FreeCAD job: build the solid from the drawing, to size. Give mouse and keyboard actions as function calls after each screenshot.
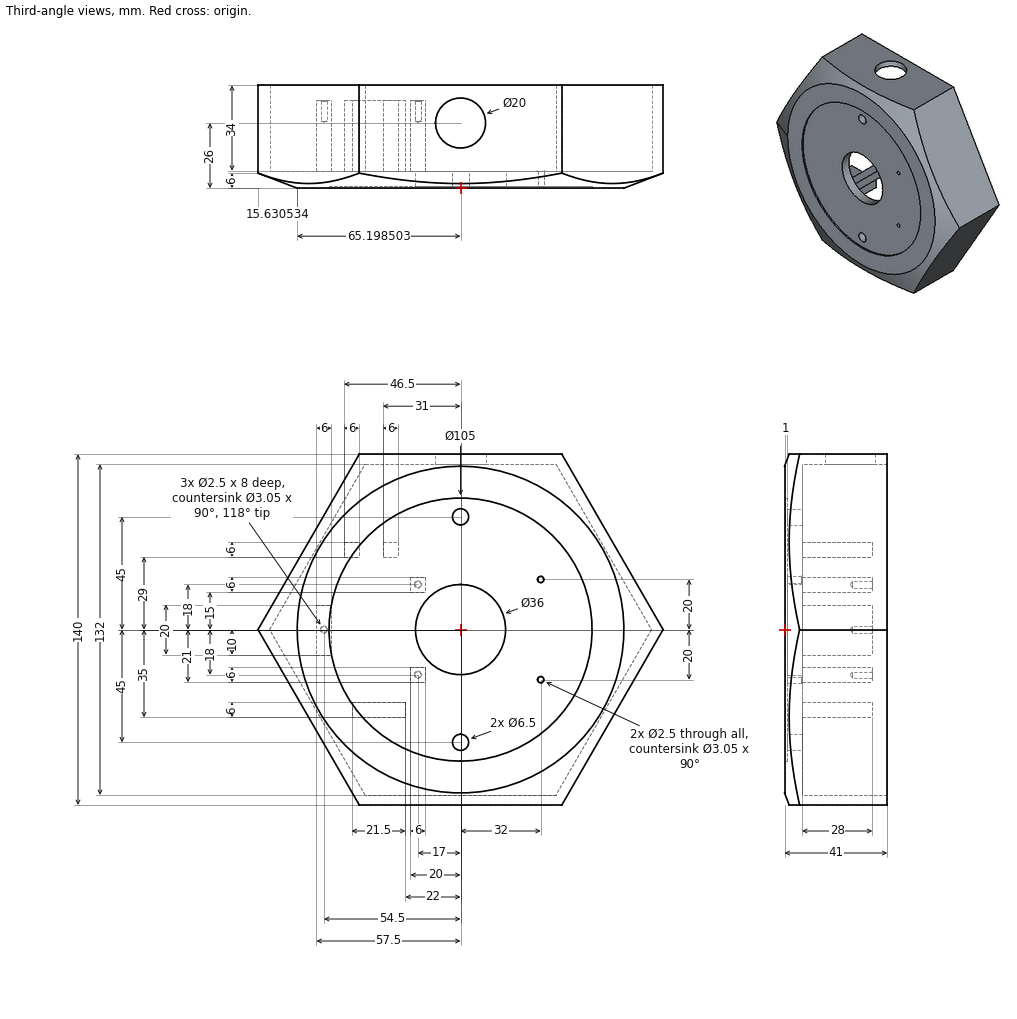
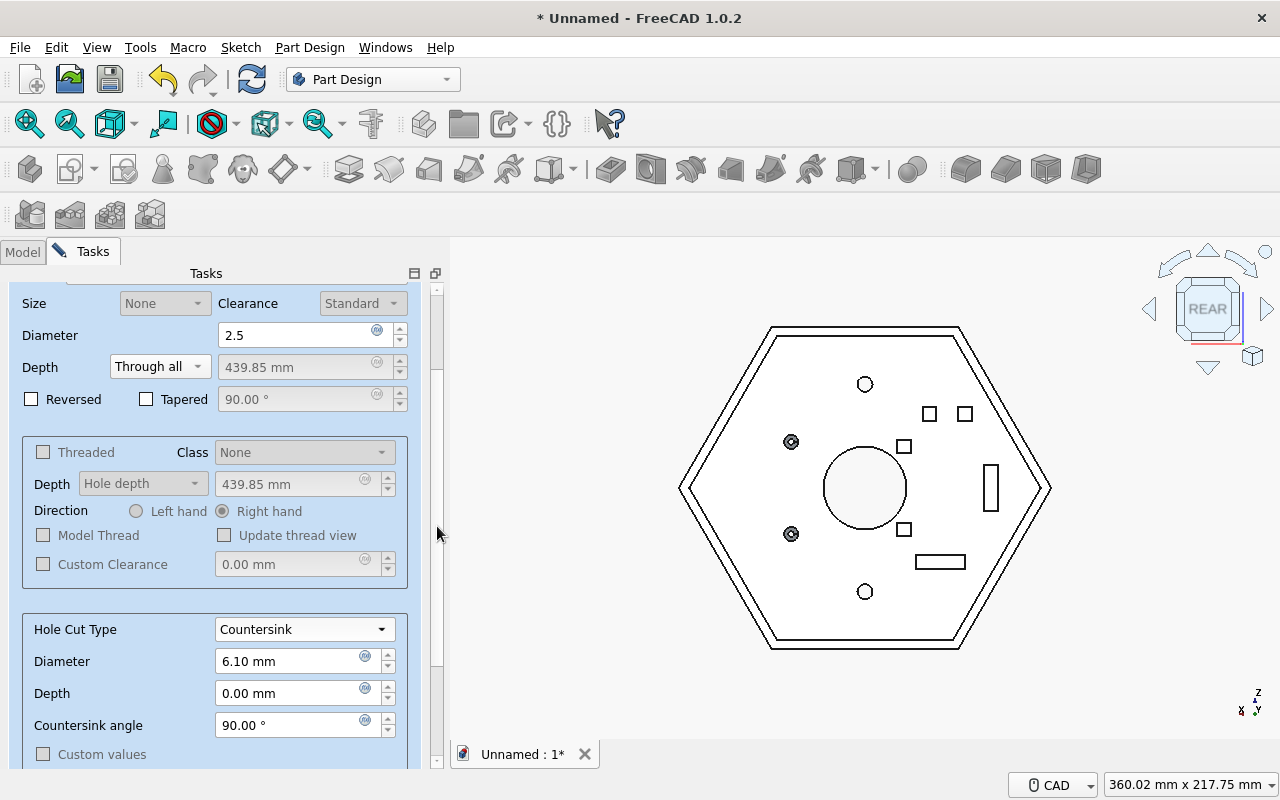
triple_click(298, 661)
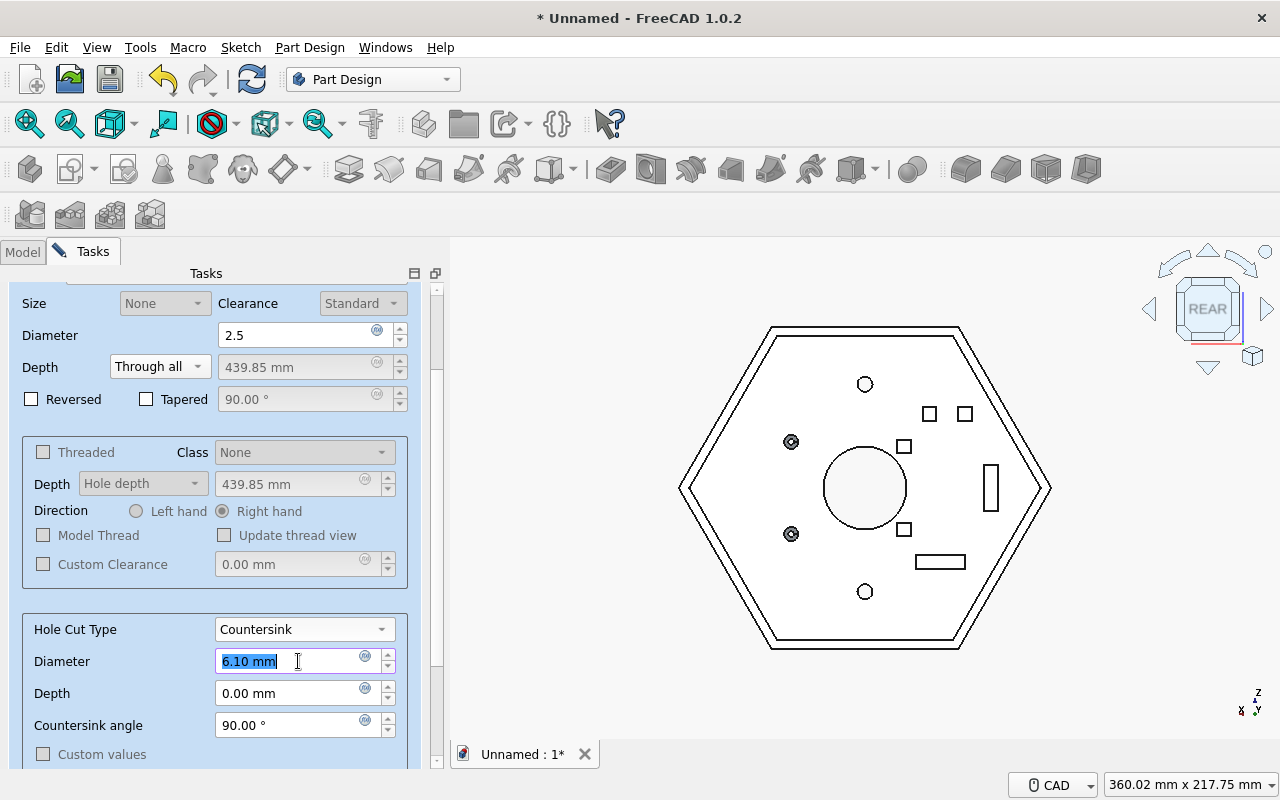
text(3.05)
key(Tab)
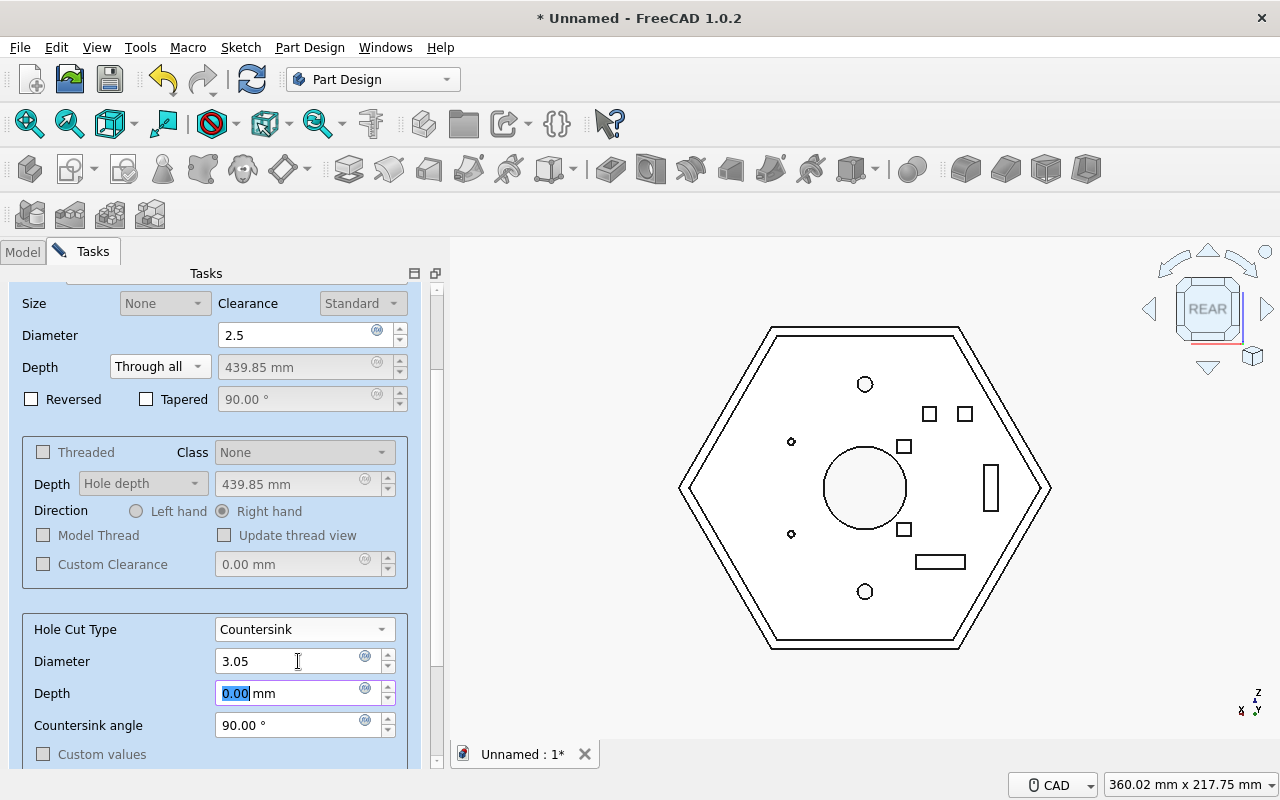
scroll(437, 526, up, 3)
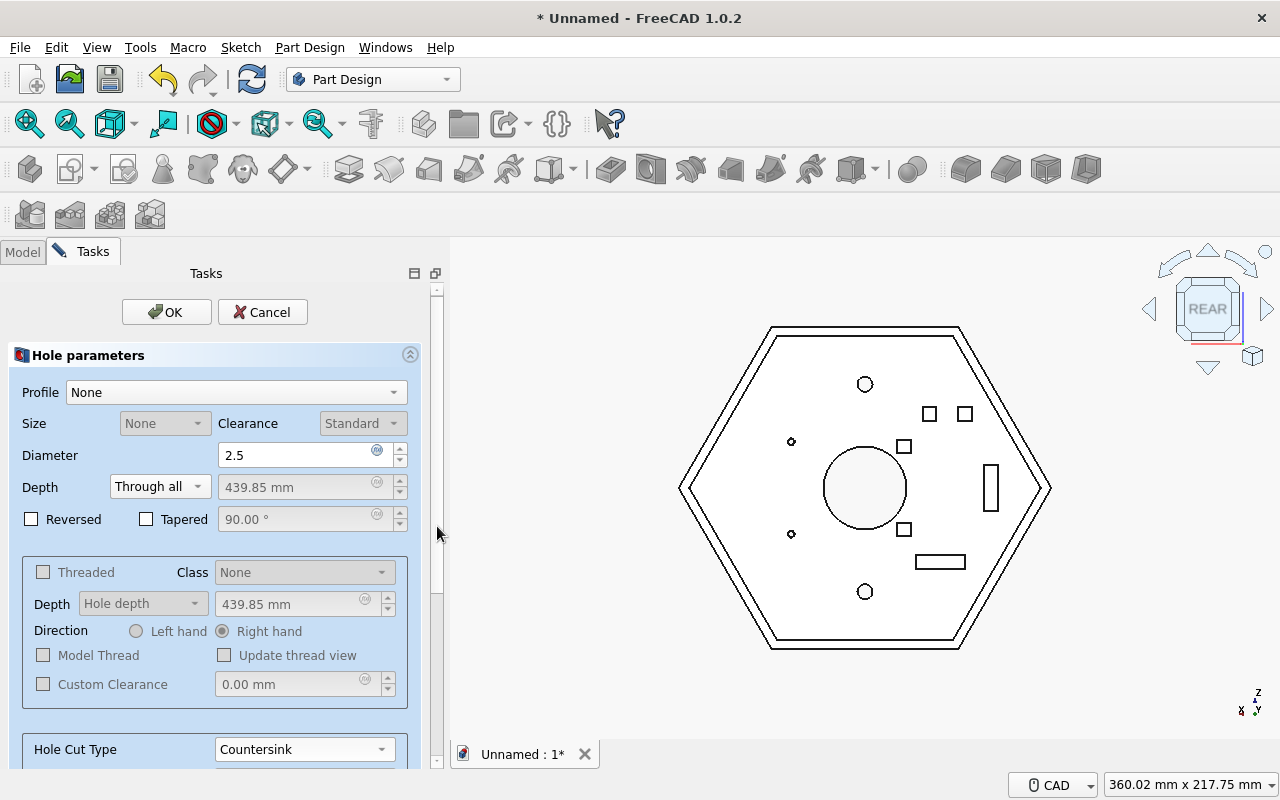
click(167, 312)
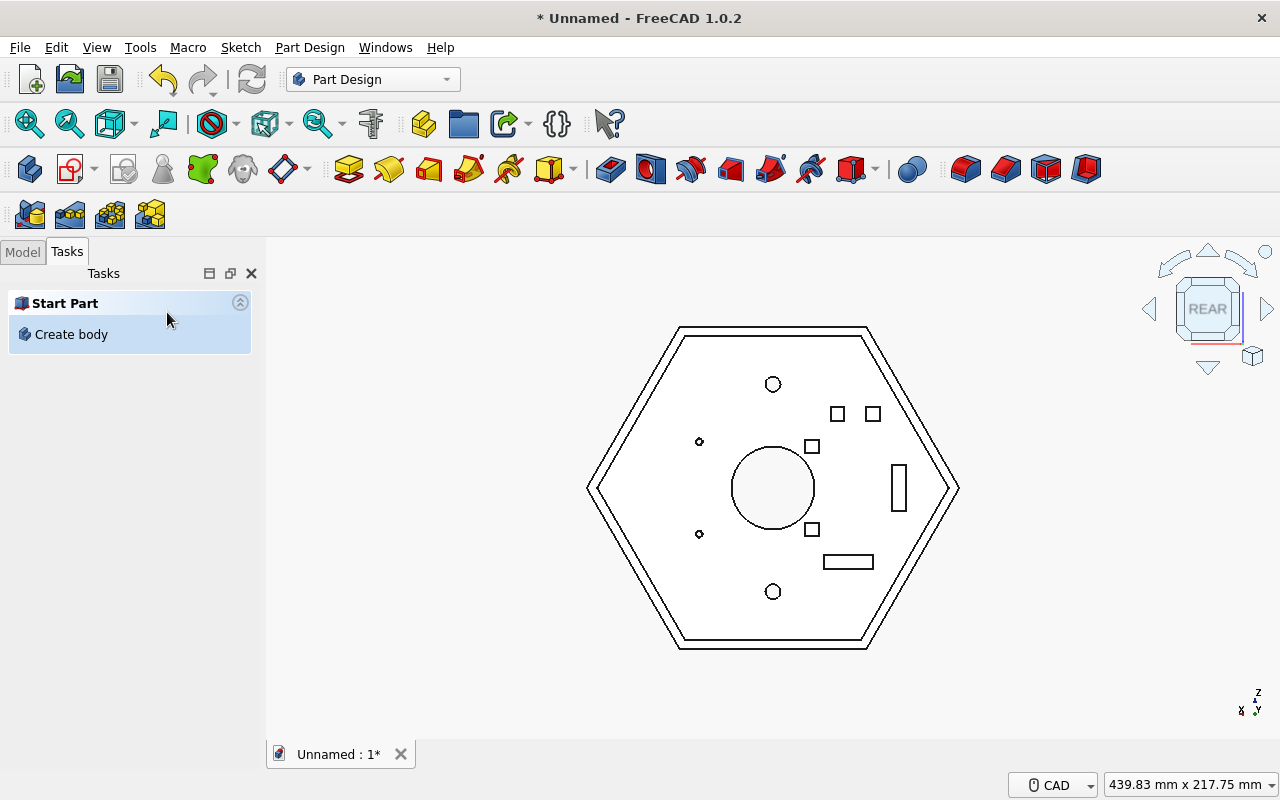
click(834, 559)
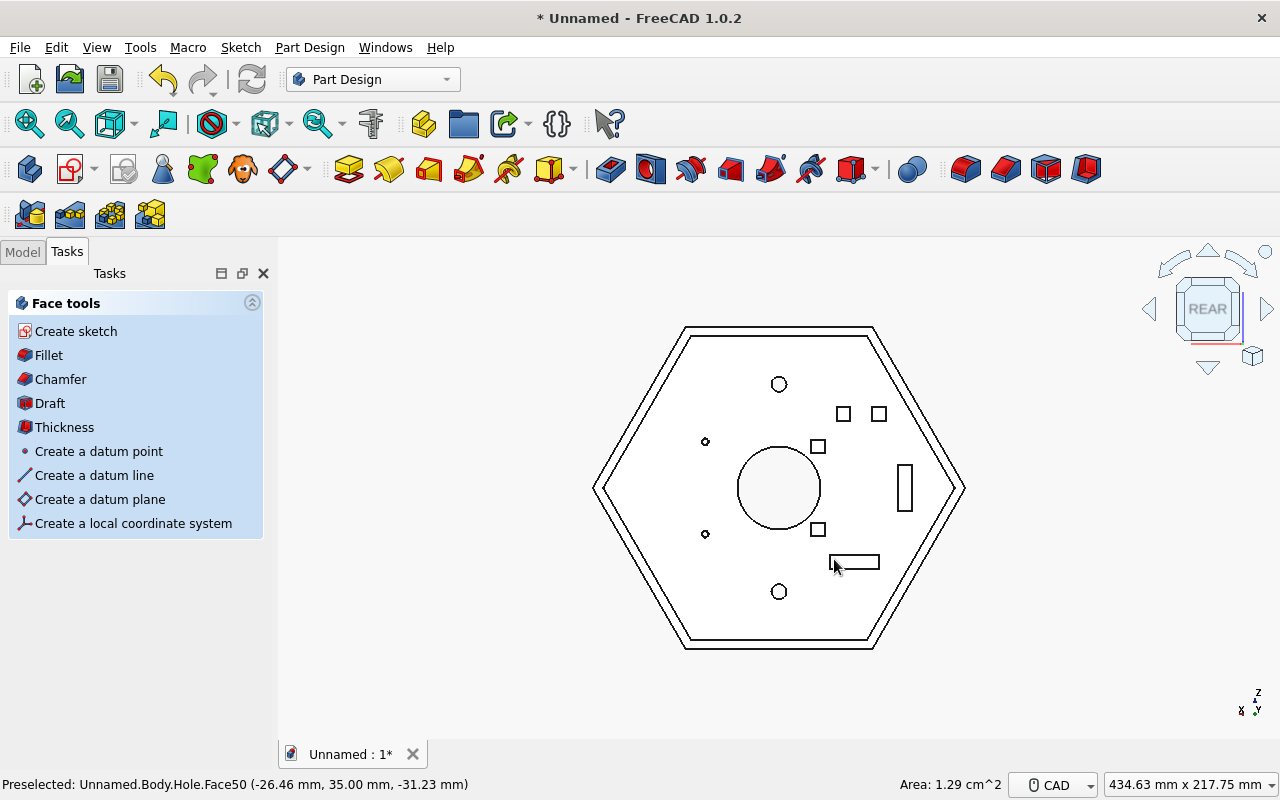
click(70, 170)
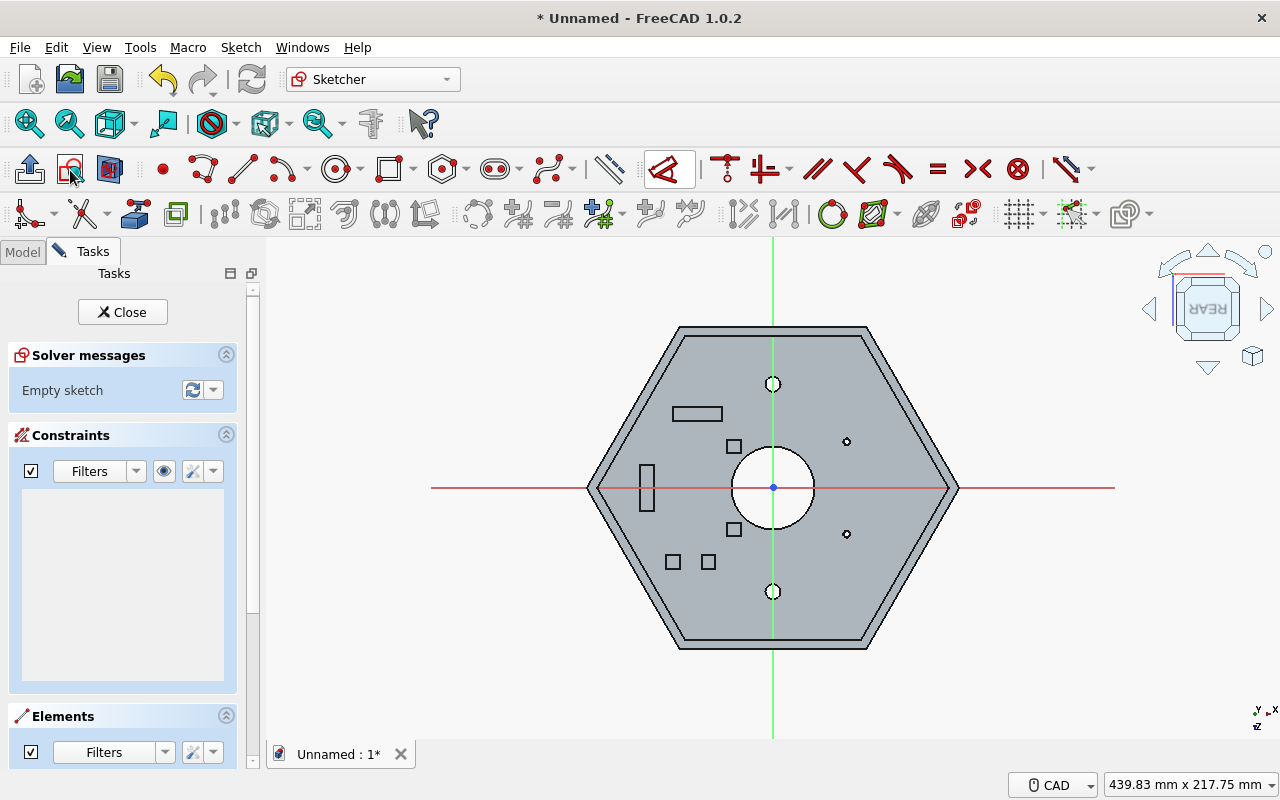
scroll(711, 488, up, 6)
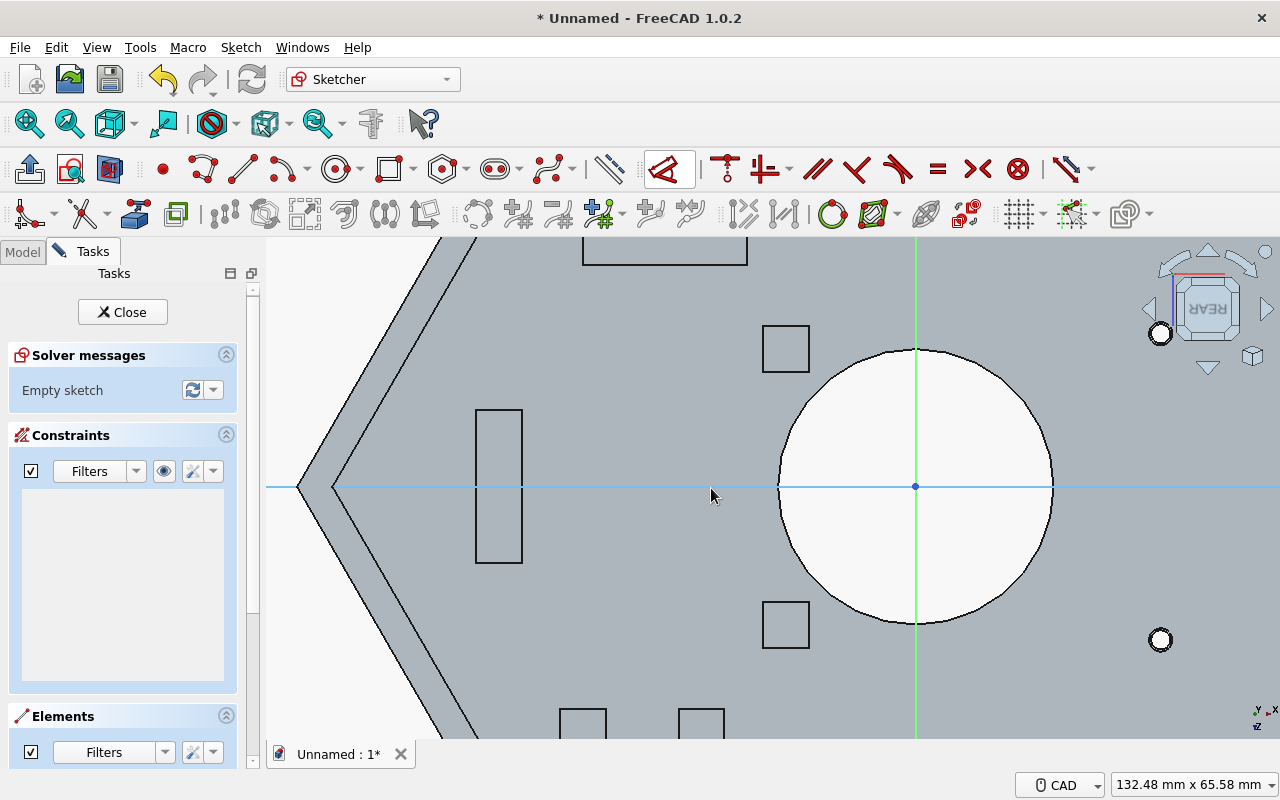
click(336, 170)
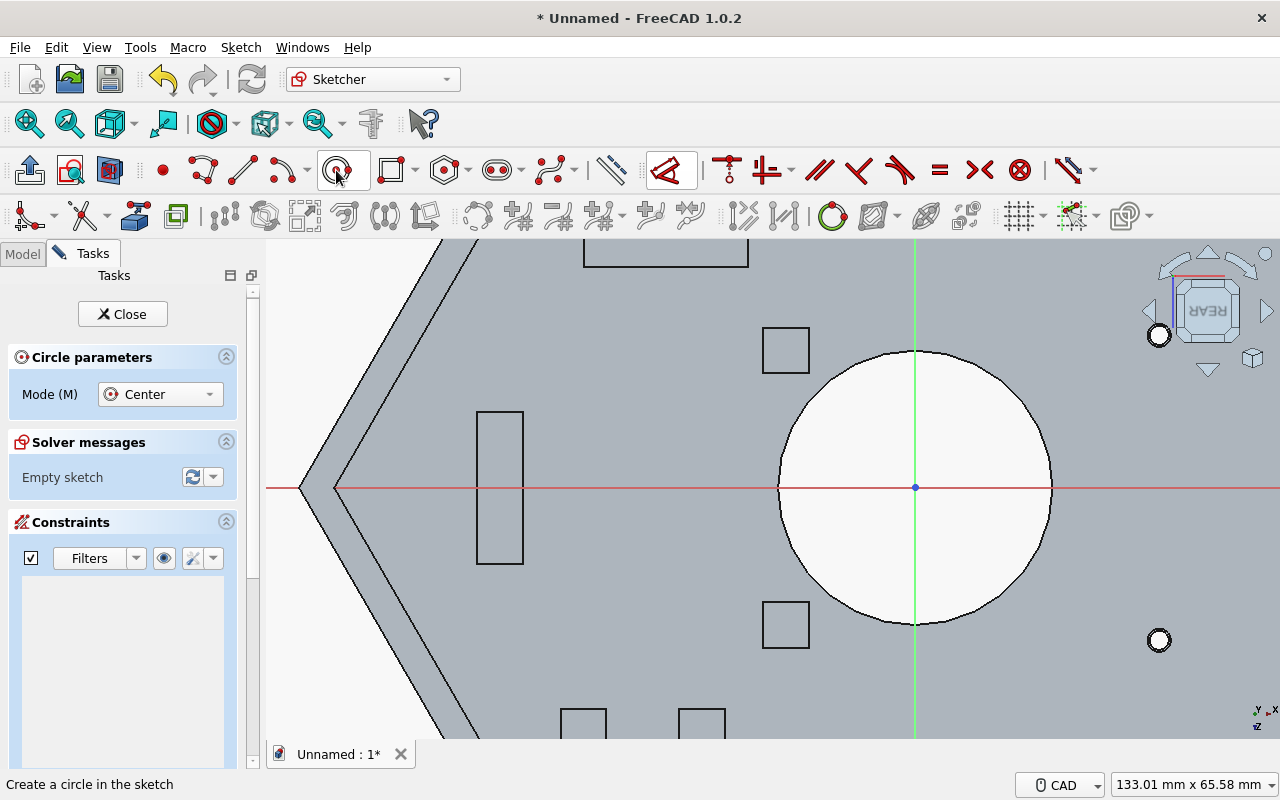
scroll(500, 488, up, 5)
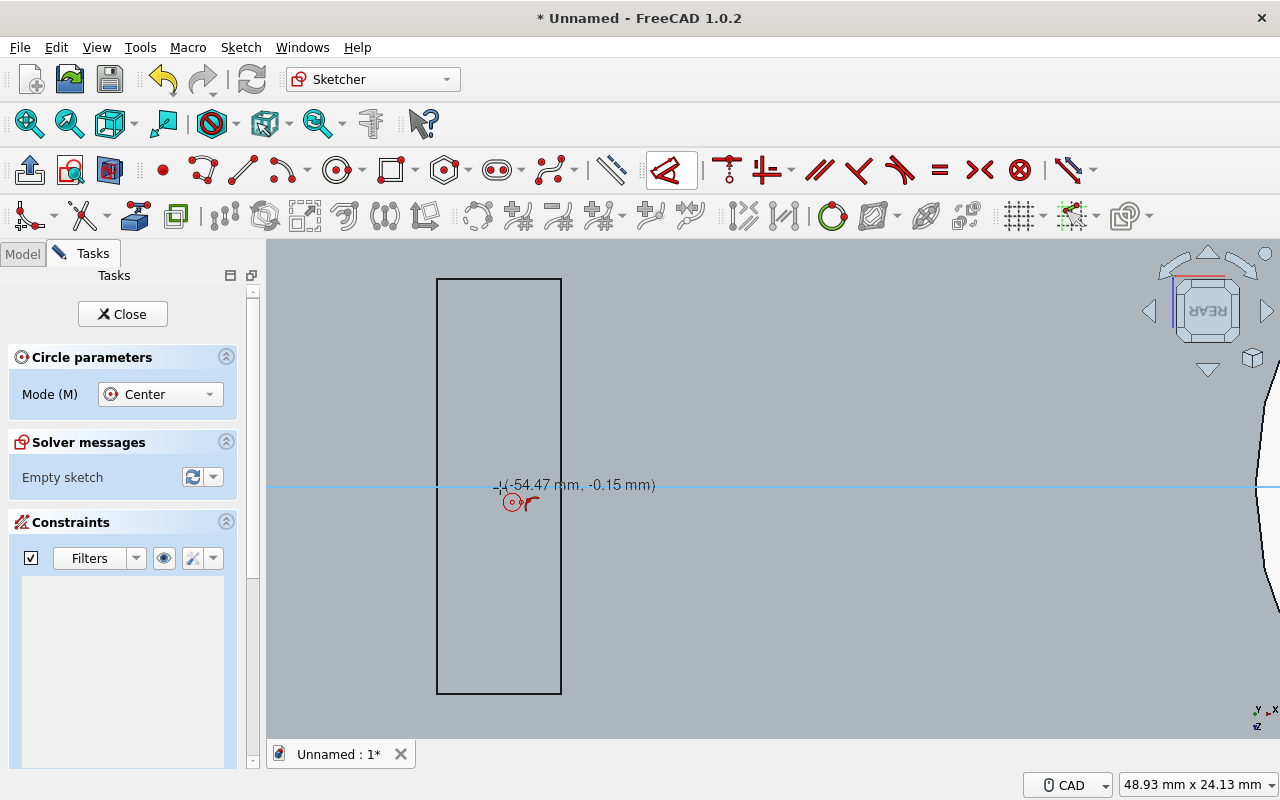
click(499, 487)
move(517, 468)